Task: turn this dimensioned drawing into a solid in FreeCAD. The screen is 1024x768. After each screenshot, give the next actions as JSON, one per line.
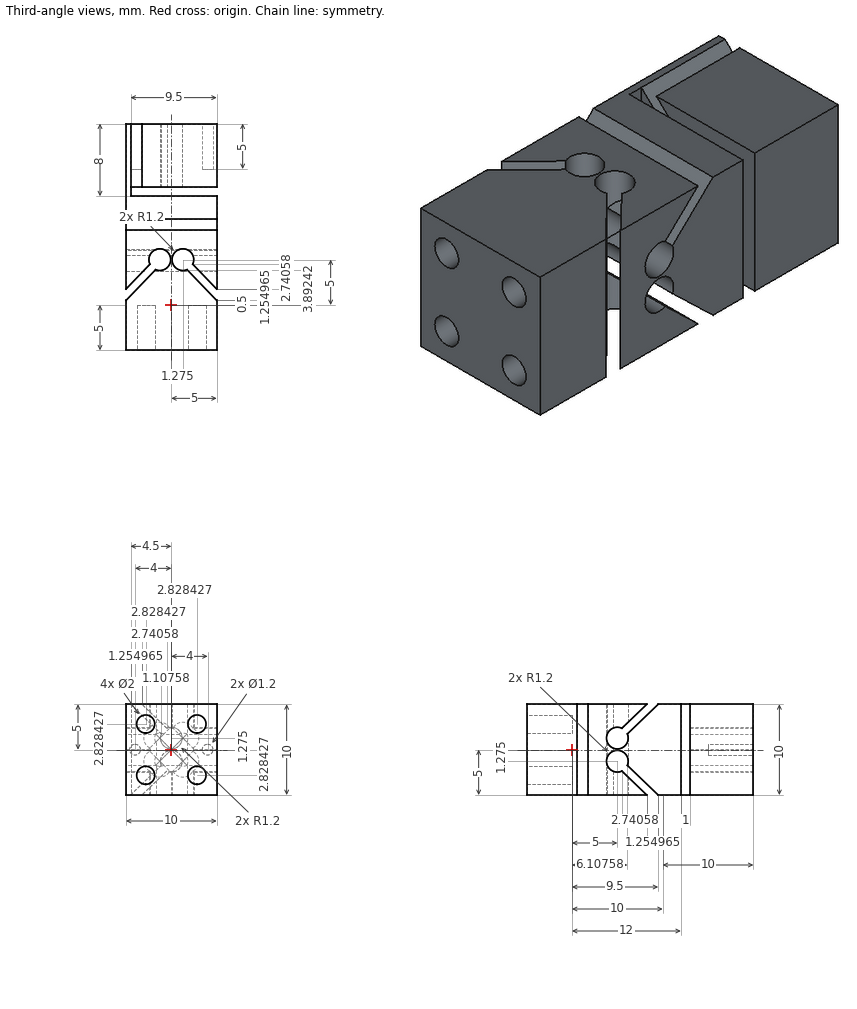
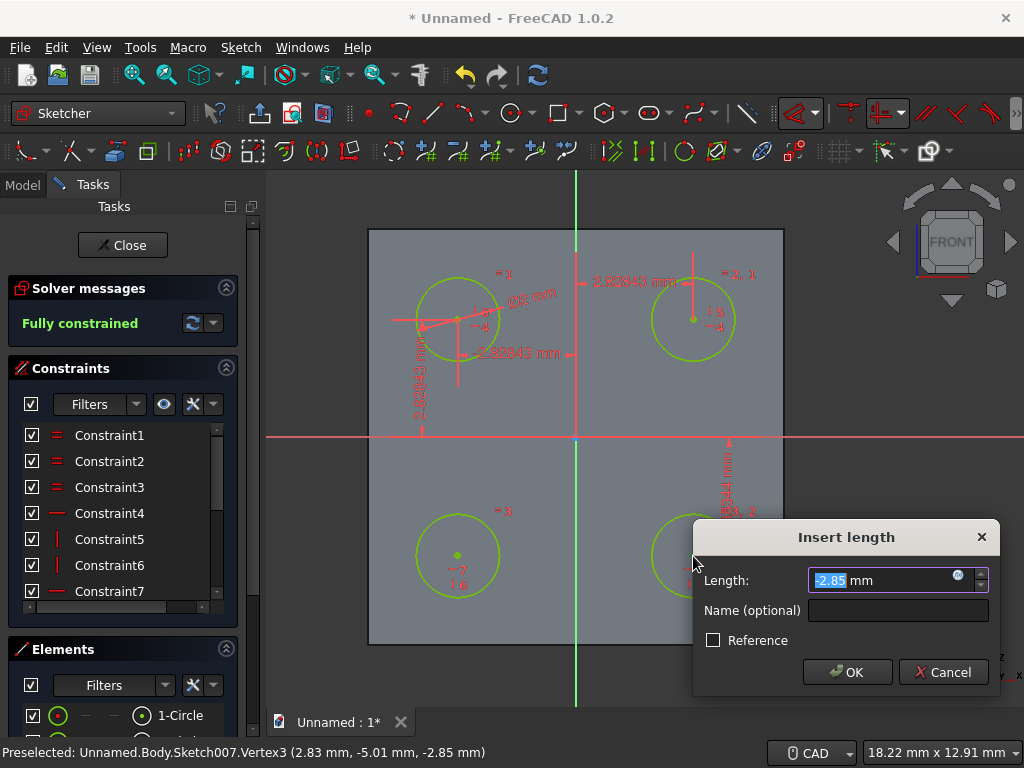
{"action": "type", "text": "-2.828427"}
{"action": "key", "text": "Return"}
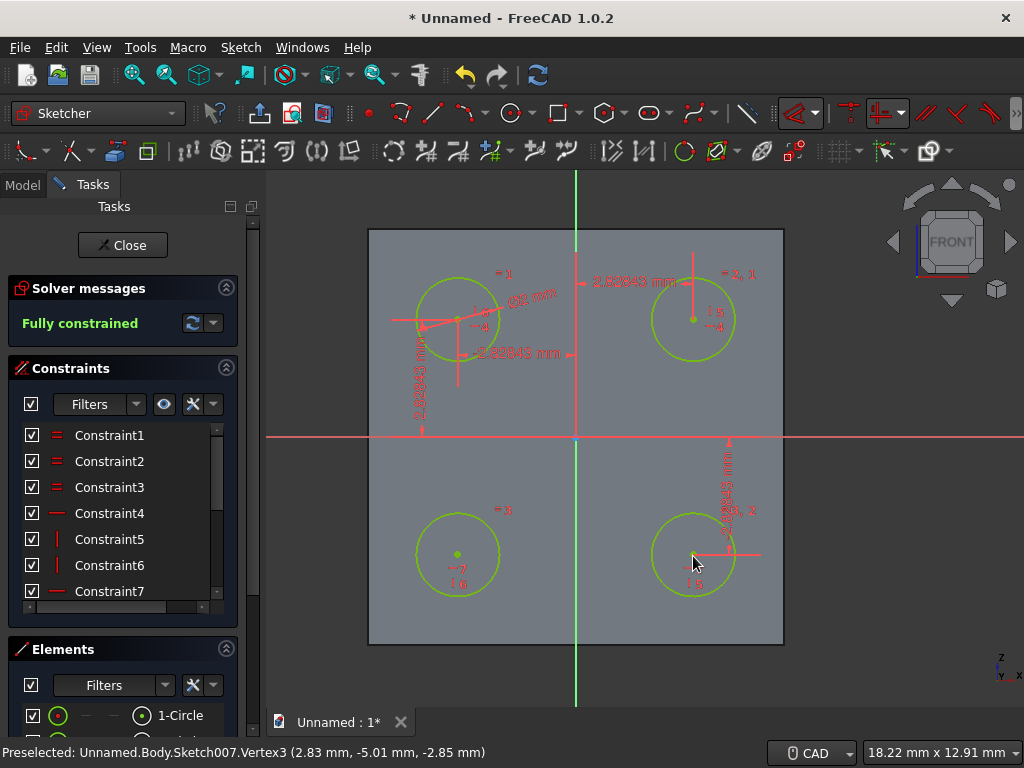
{"action": "left_click", "coordinate": [123, 245]}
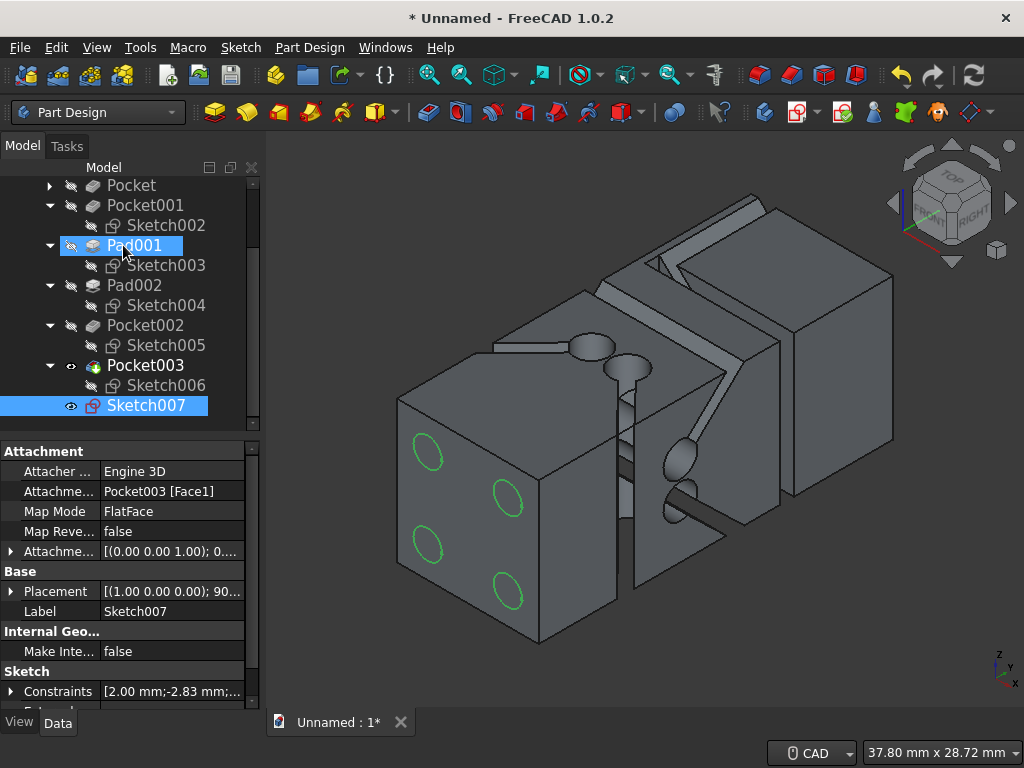
{"action": "left_click", "coordinate": [430, 112]}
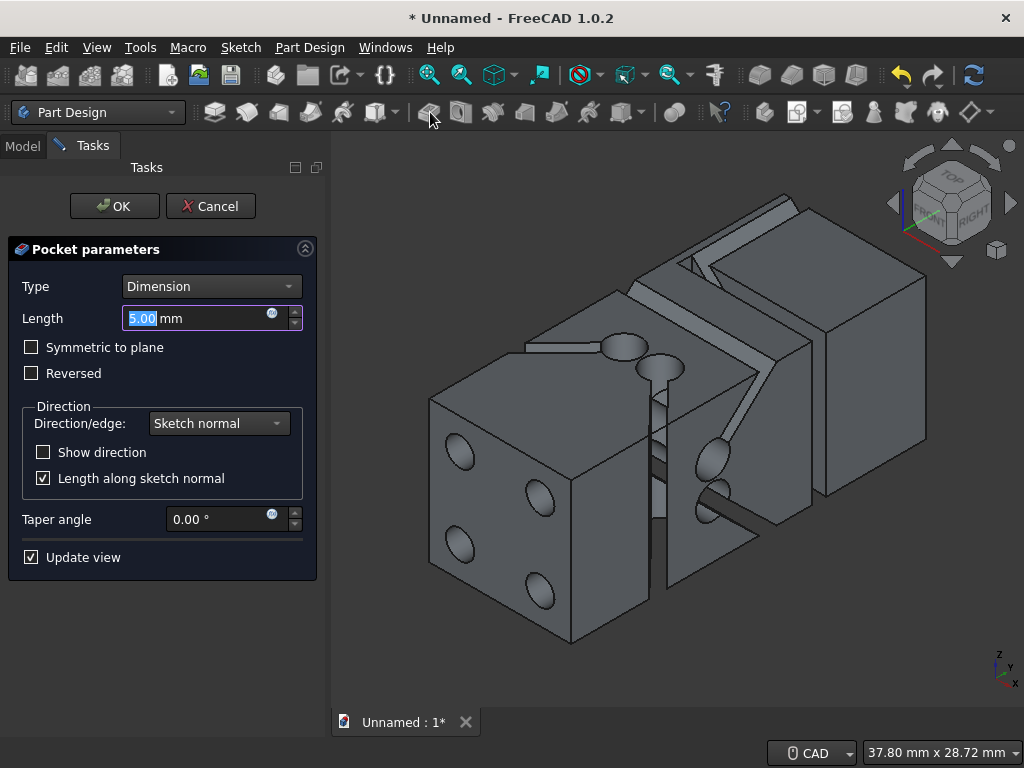
{"action": "type", "text": "5"}
{"action": "key", "text": "Tab"}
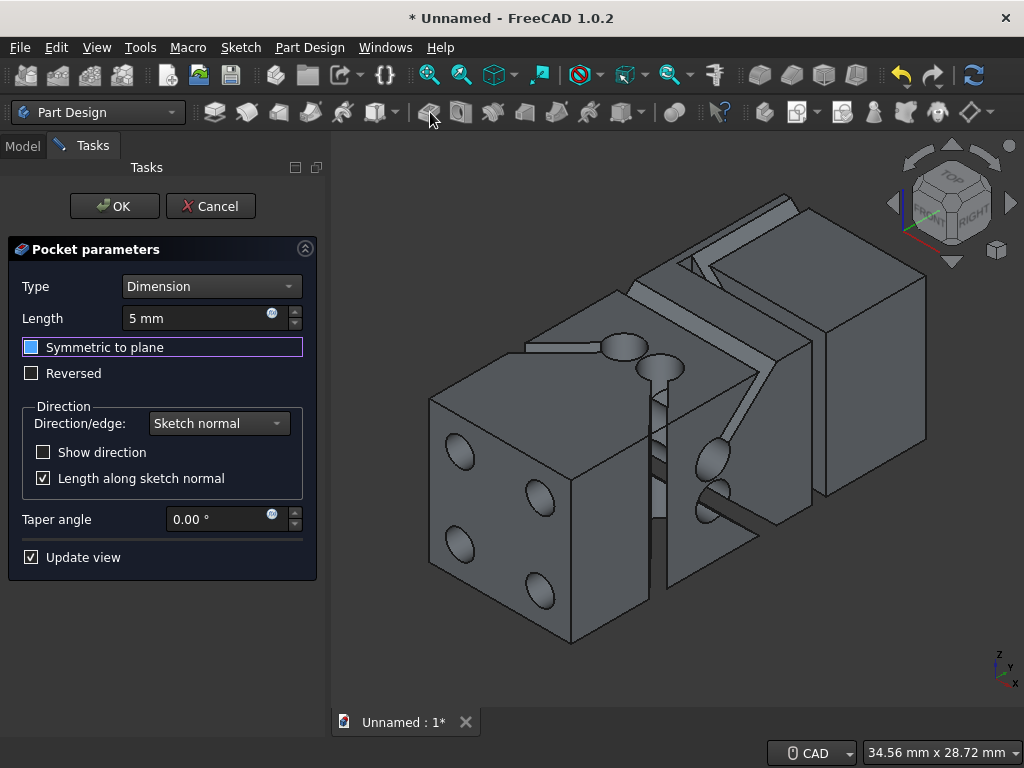
{"action": "left_click", "coordinate": [115, 206]}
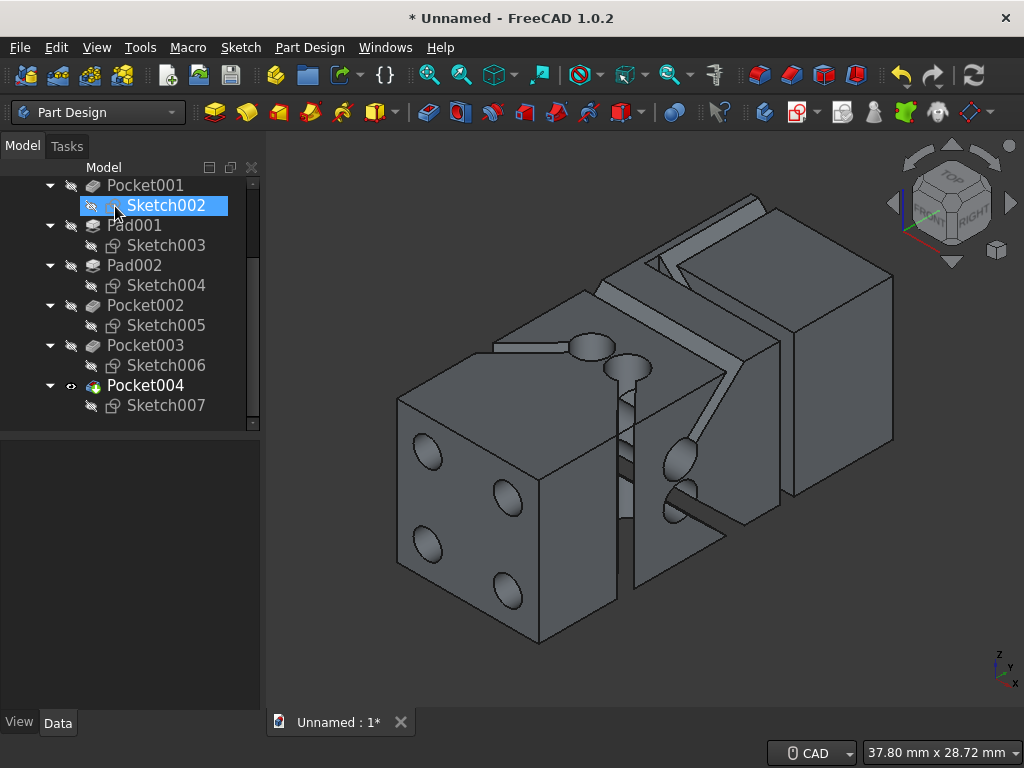
{"action": "key", "text": "4"}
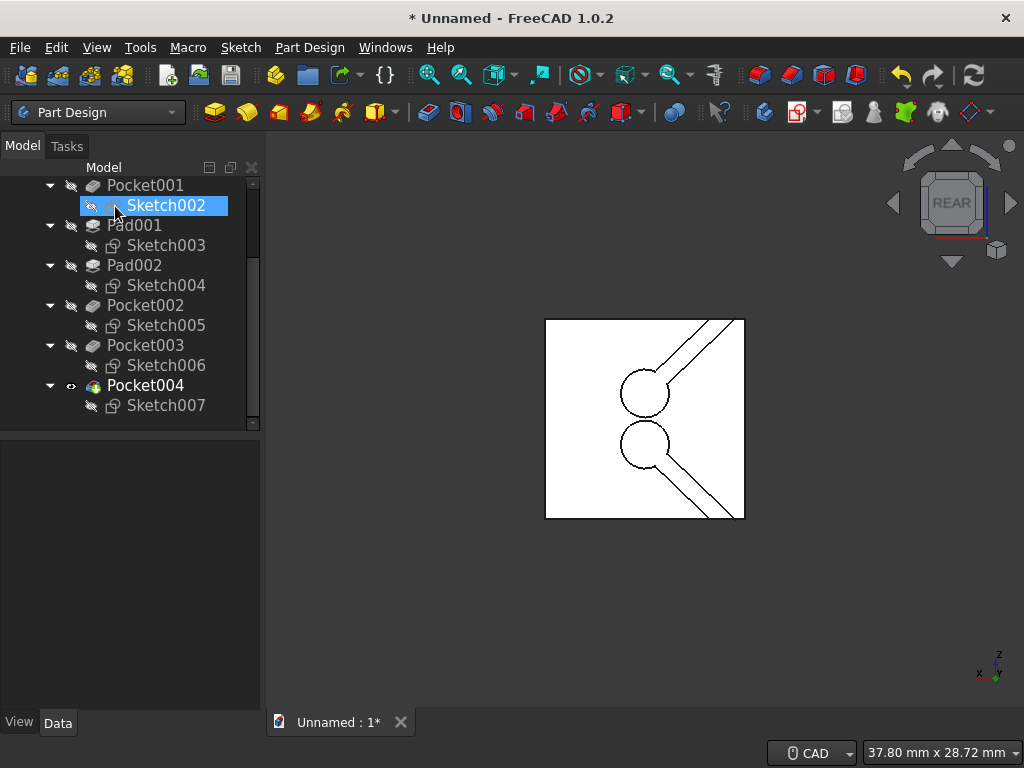
{"action": "left_click", "coordinate": [430, 76]}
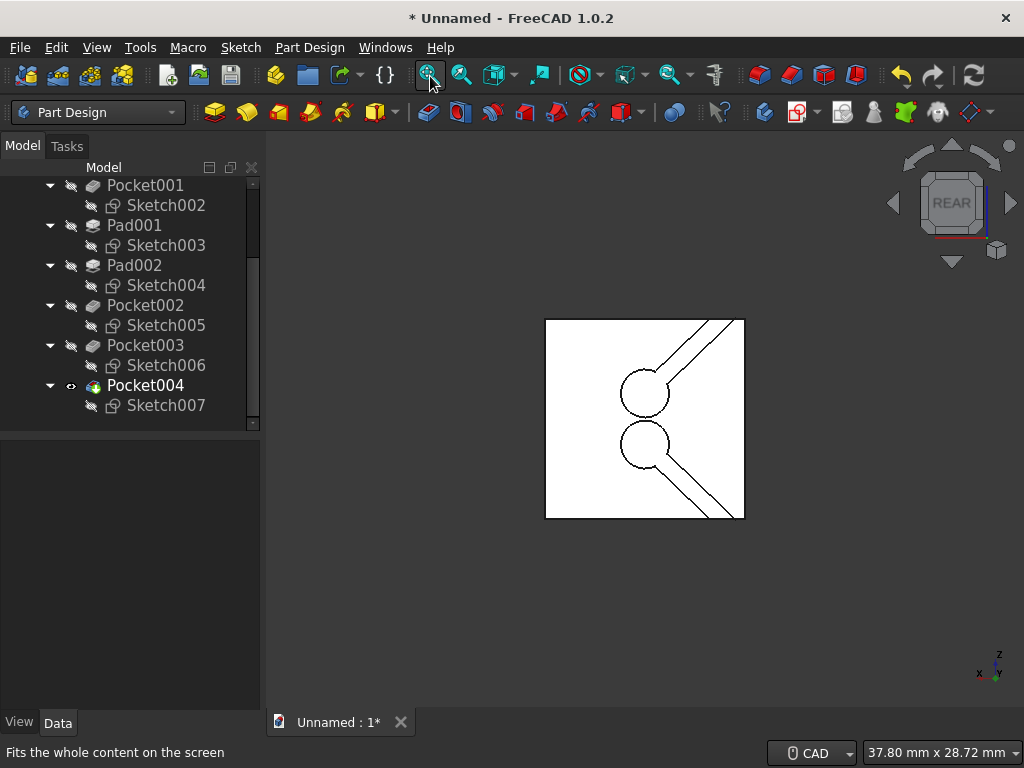
{"action": "left_click", "coordinate": [588, 475]}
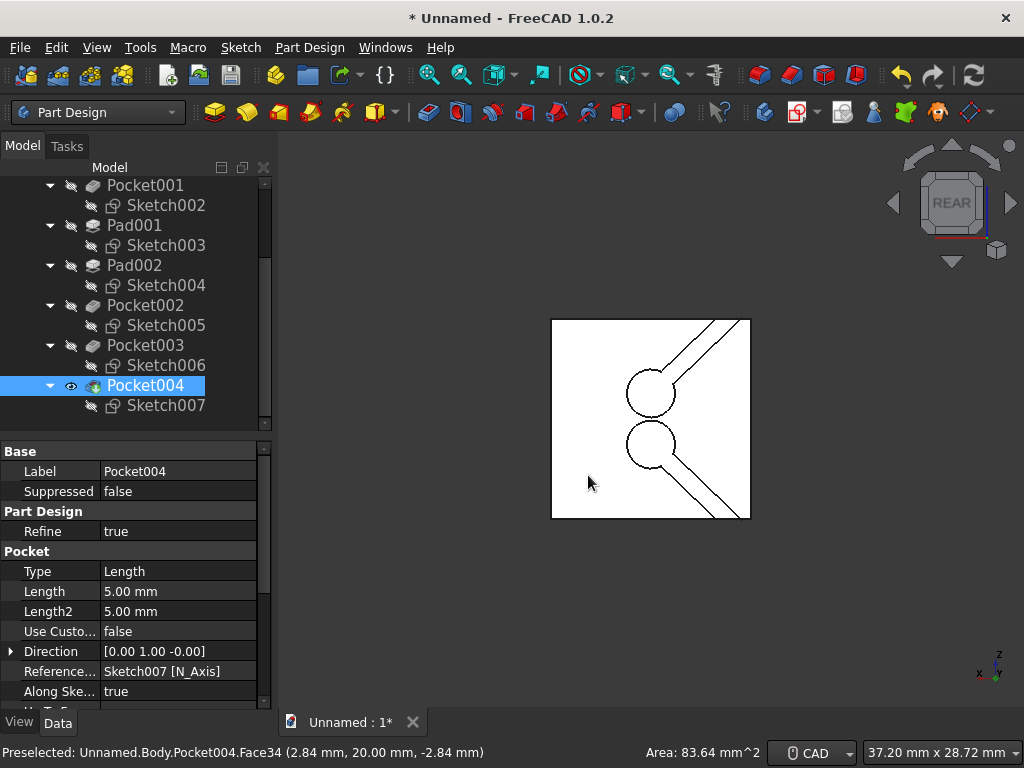
{"action": "left_click", "coordinate": [798, 112]}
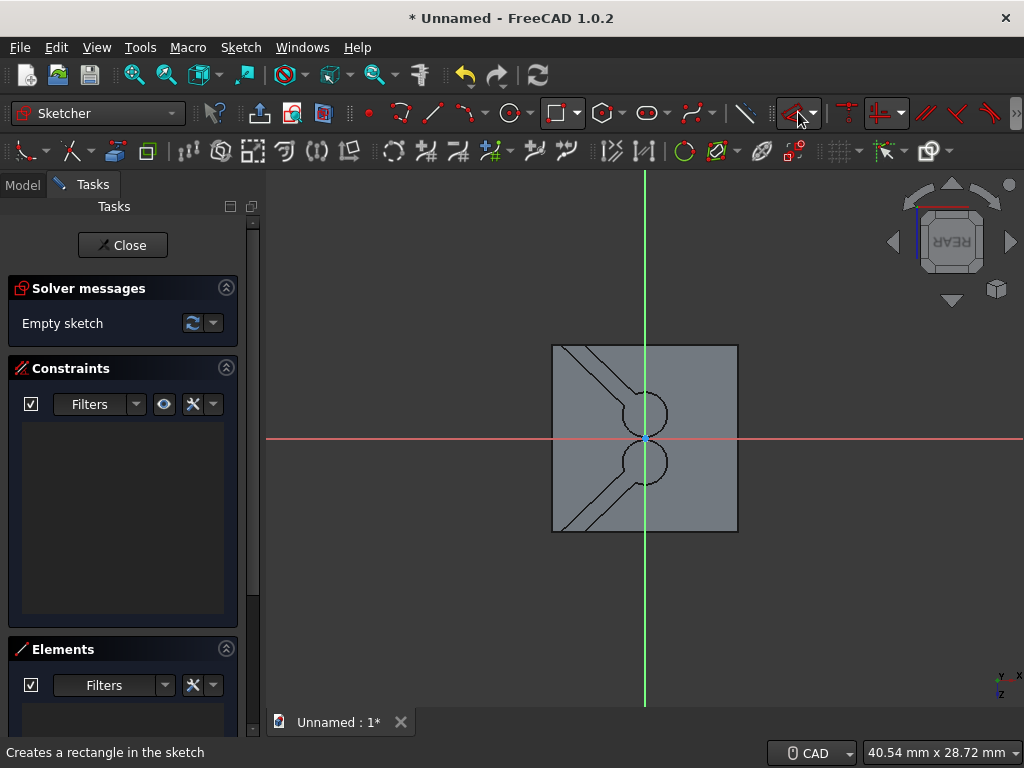
{"action": "scroll", "coordinate": [701, 438], "scroll_direction": "up", "scroll_amount": 4}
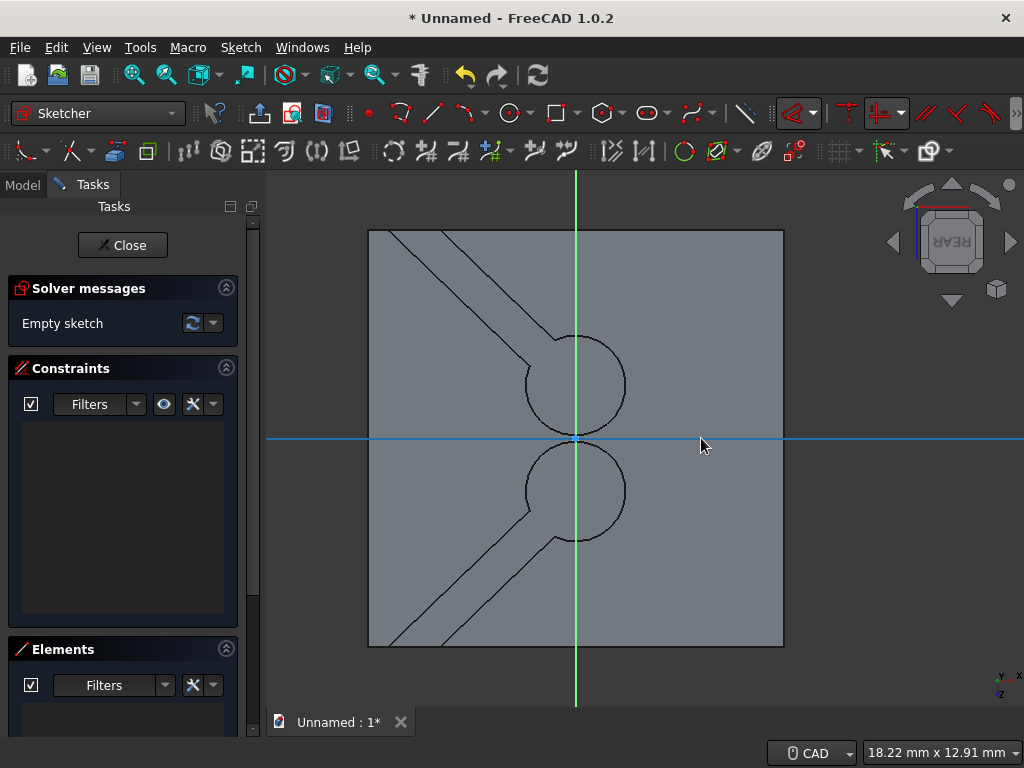
{"action": "key", "text": "g c"}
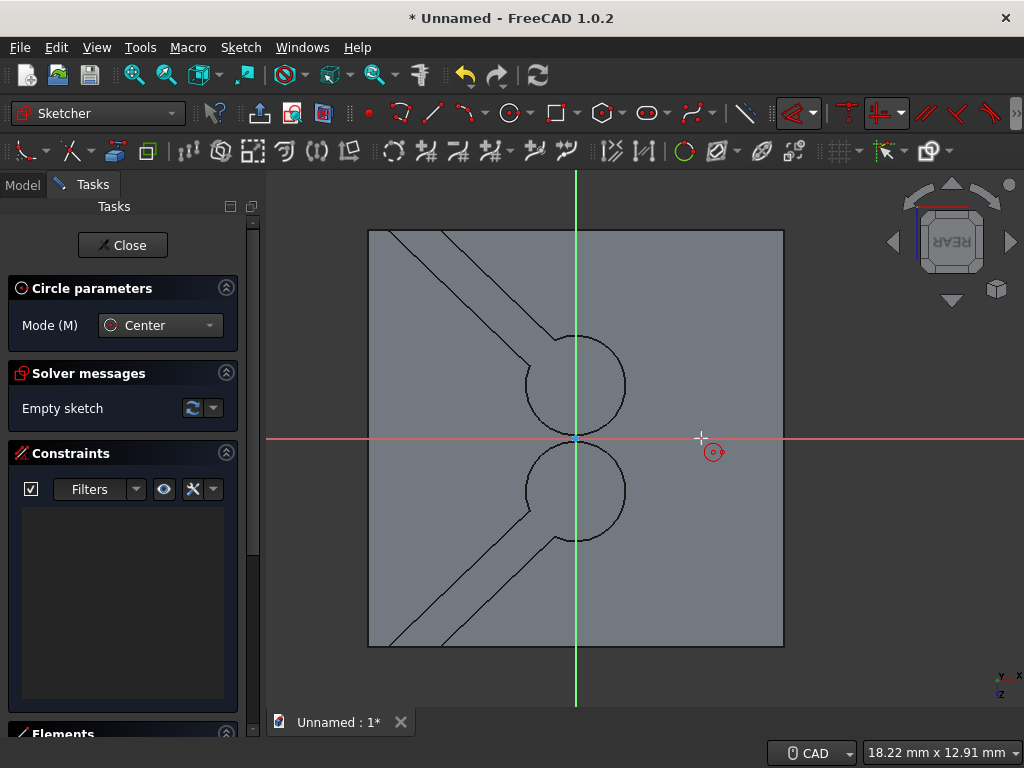
{"action": "left_click", "coordinate": [742, 438]}
{"action": "left_click", "coordinate": [760, 421]}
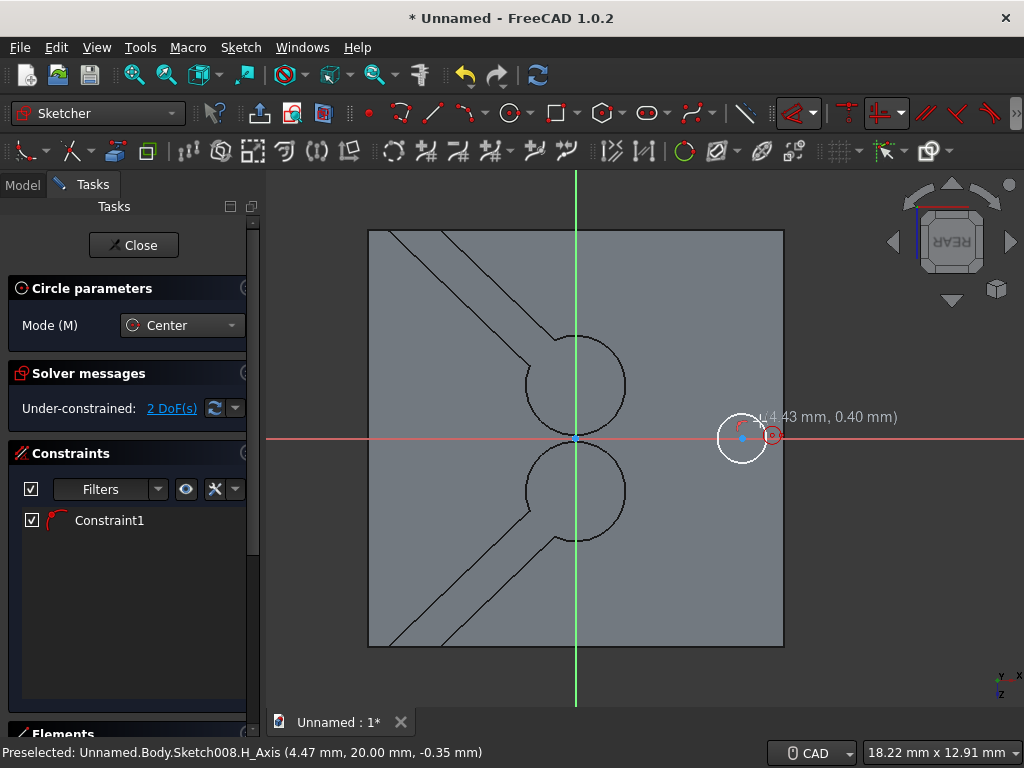
{"action": "left_click", "coordinate": [409, 438]}
{"action": "left_click", "coordinate": [427, 421]}
{"action": "key", "text": "Escape"}